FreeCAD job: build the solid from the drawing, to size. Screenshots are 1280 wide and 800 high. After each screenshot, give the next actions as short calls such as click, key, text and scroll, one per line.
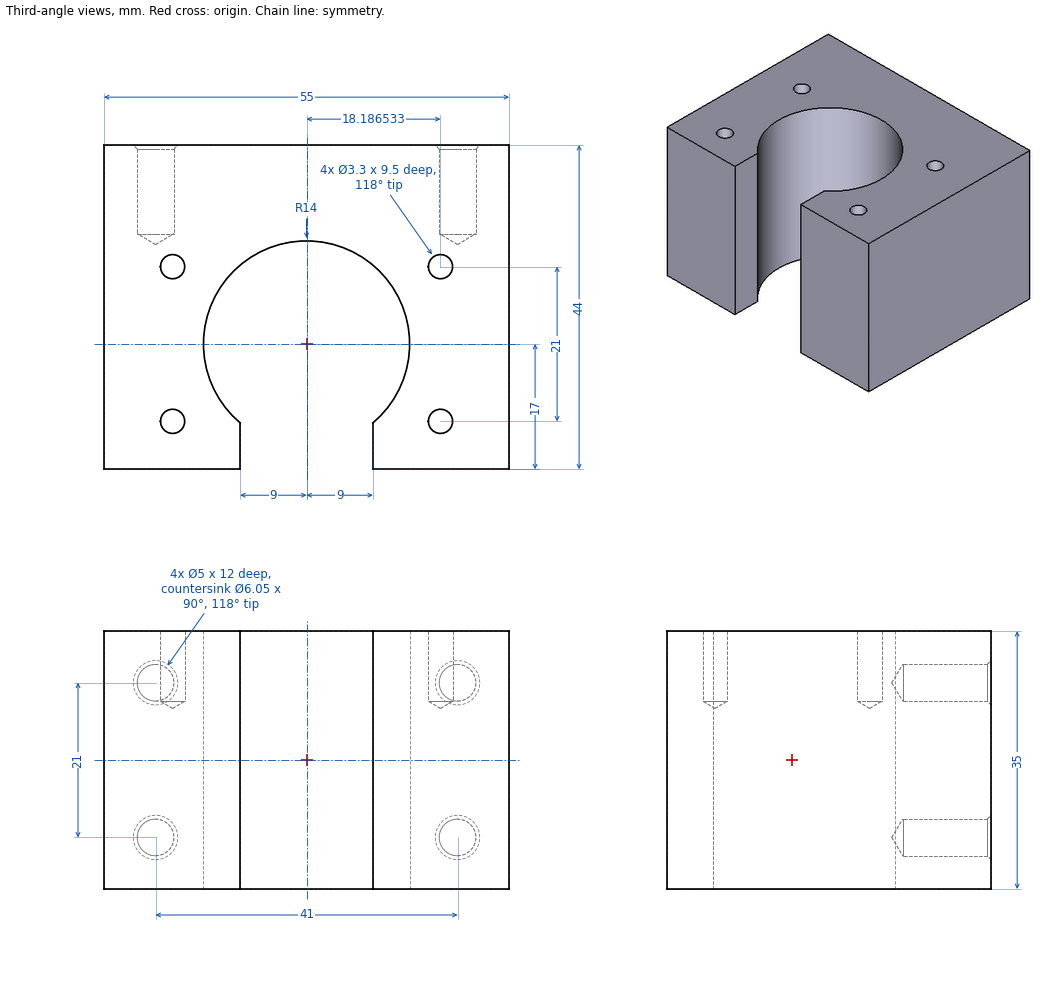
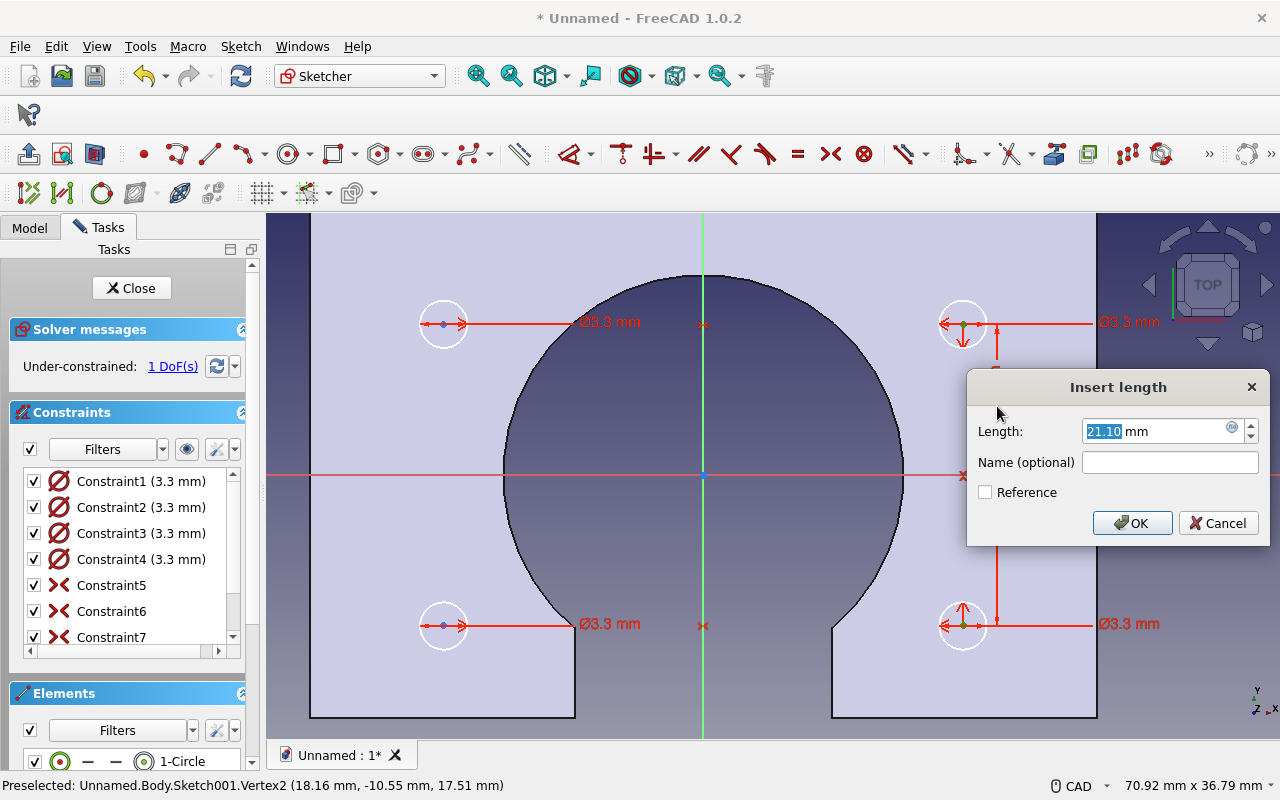
text(21)
key(Return)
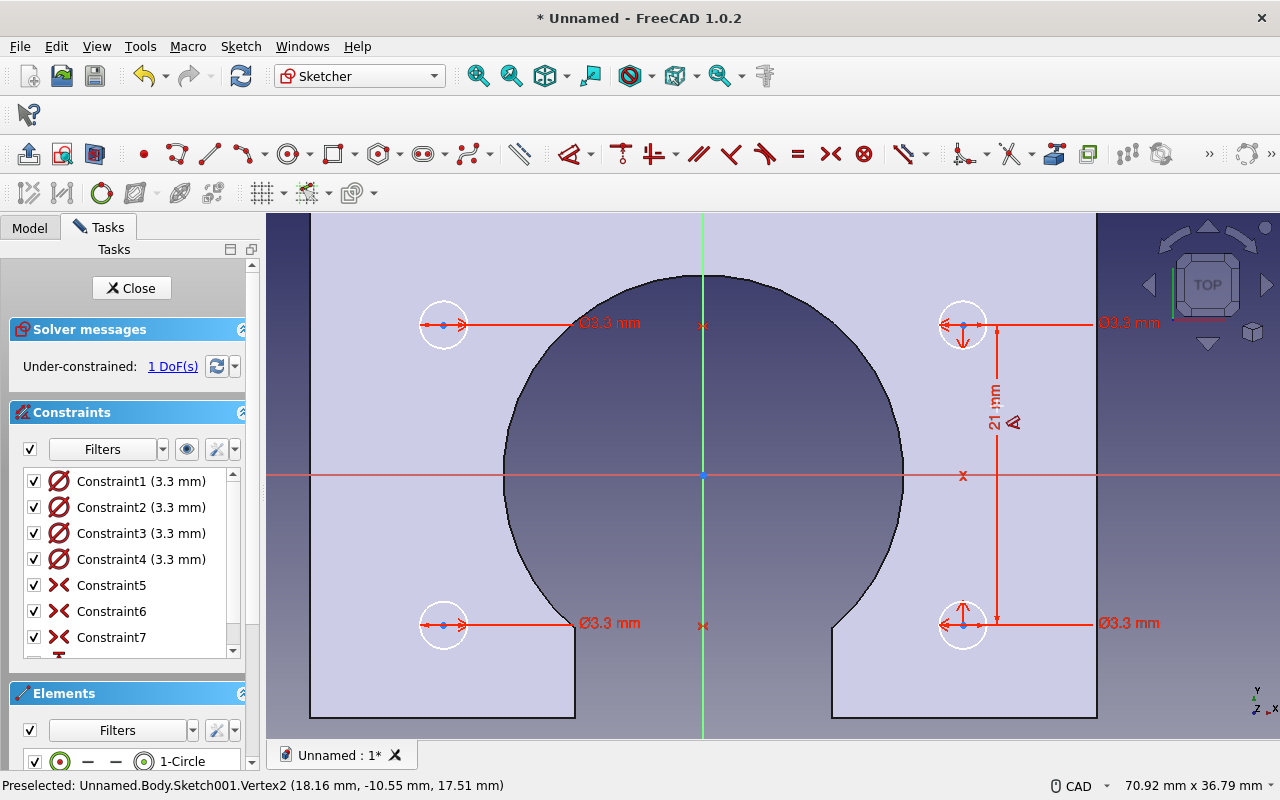
click(963, 325)
click(833, 291)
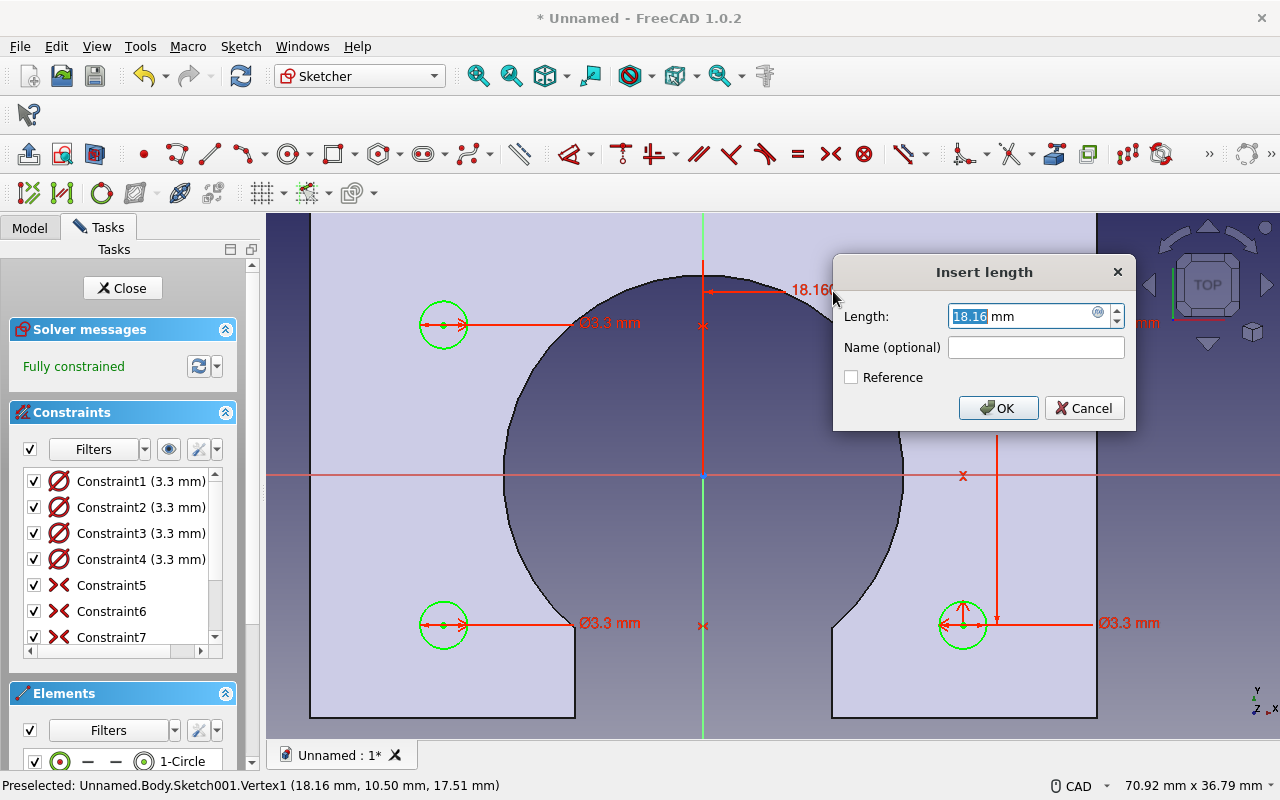
text(18.186533)
key(Return)
key(Escape)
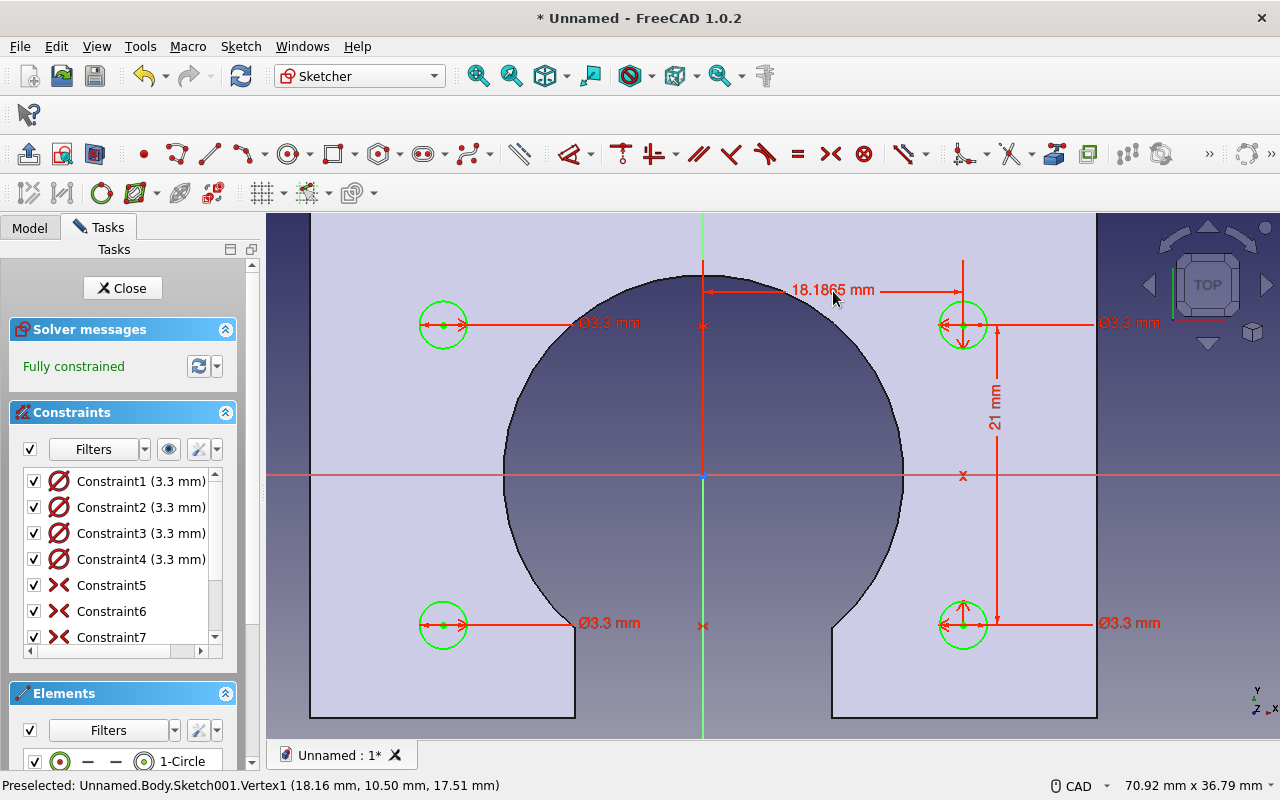
click(123, 288)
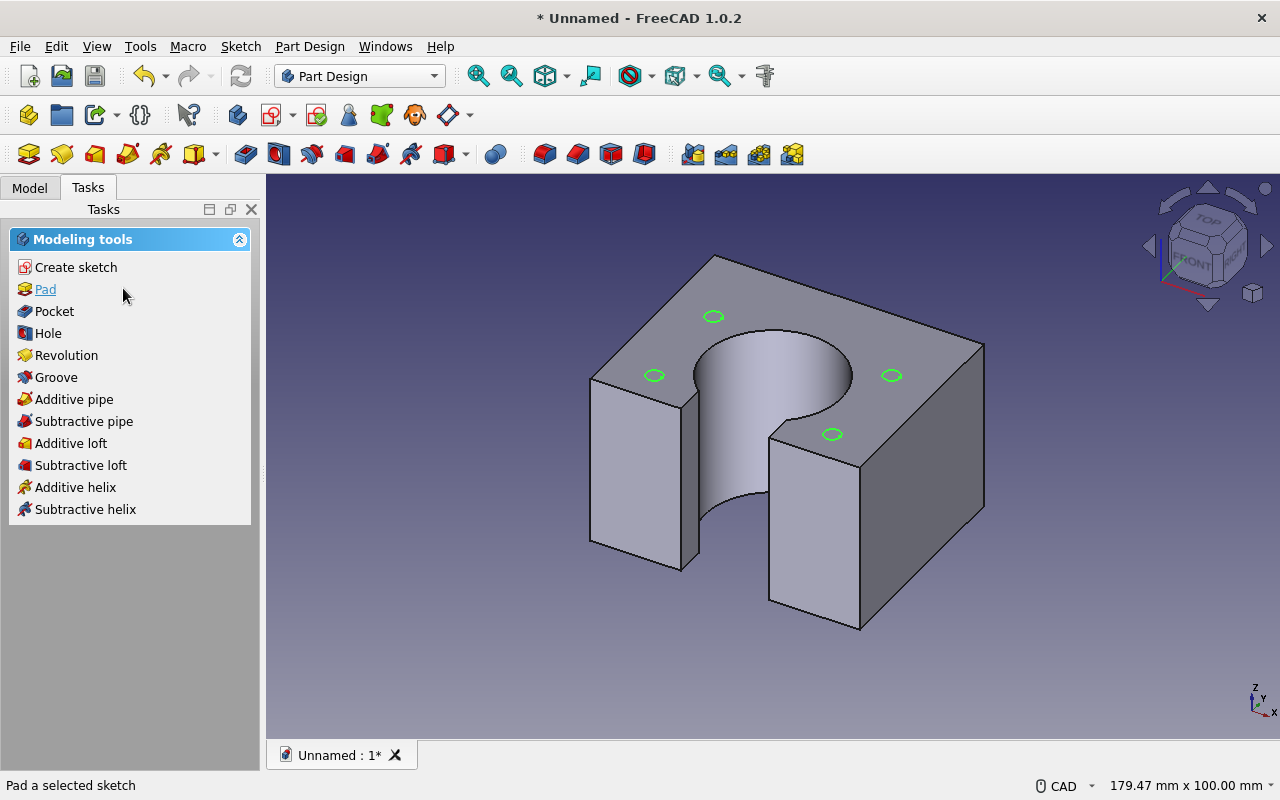
click(279, 154)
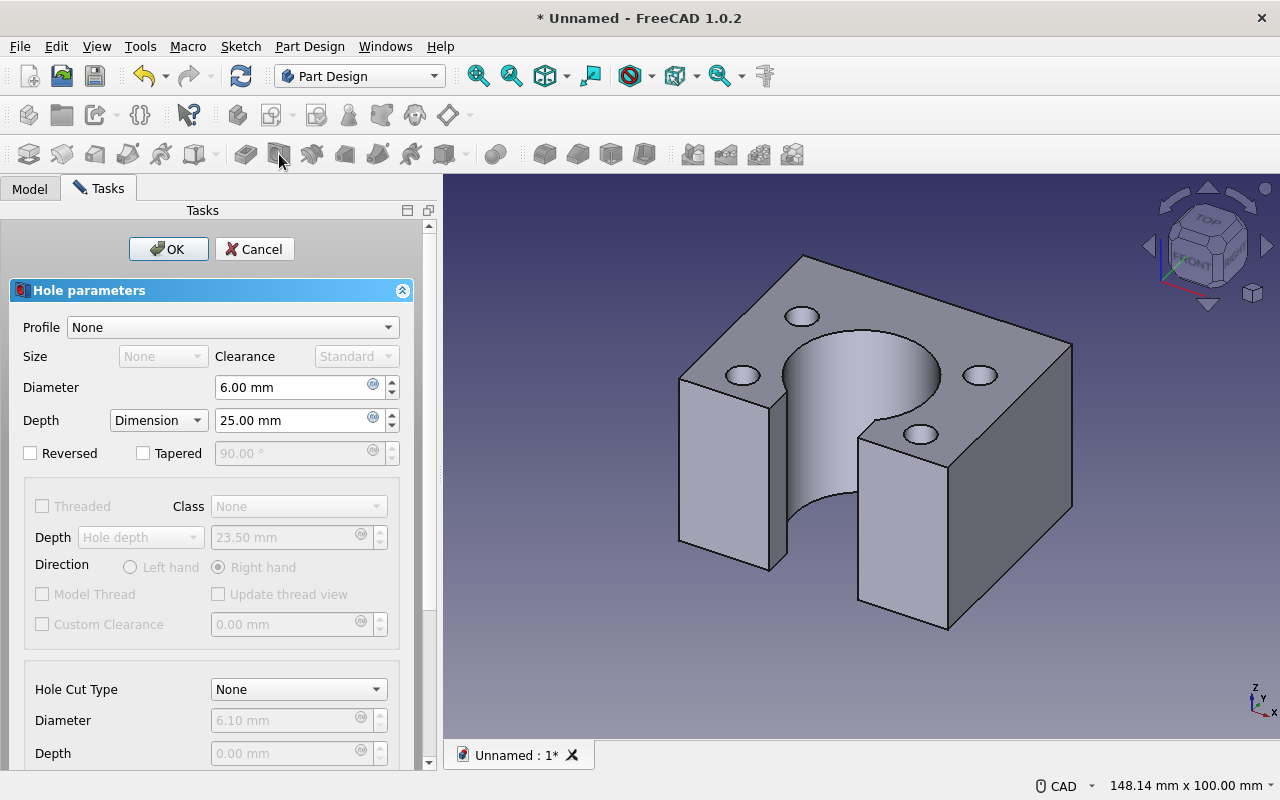
triple_click(300, 388)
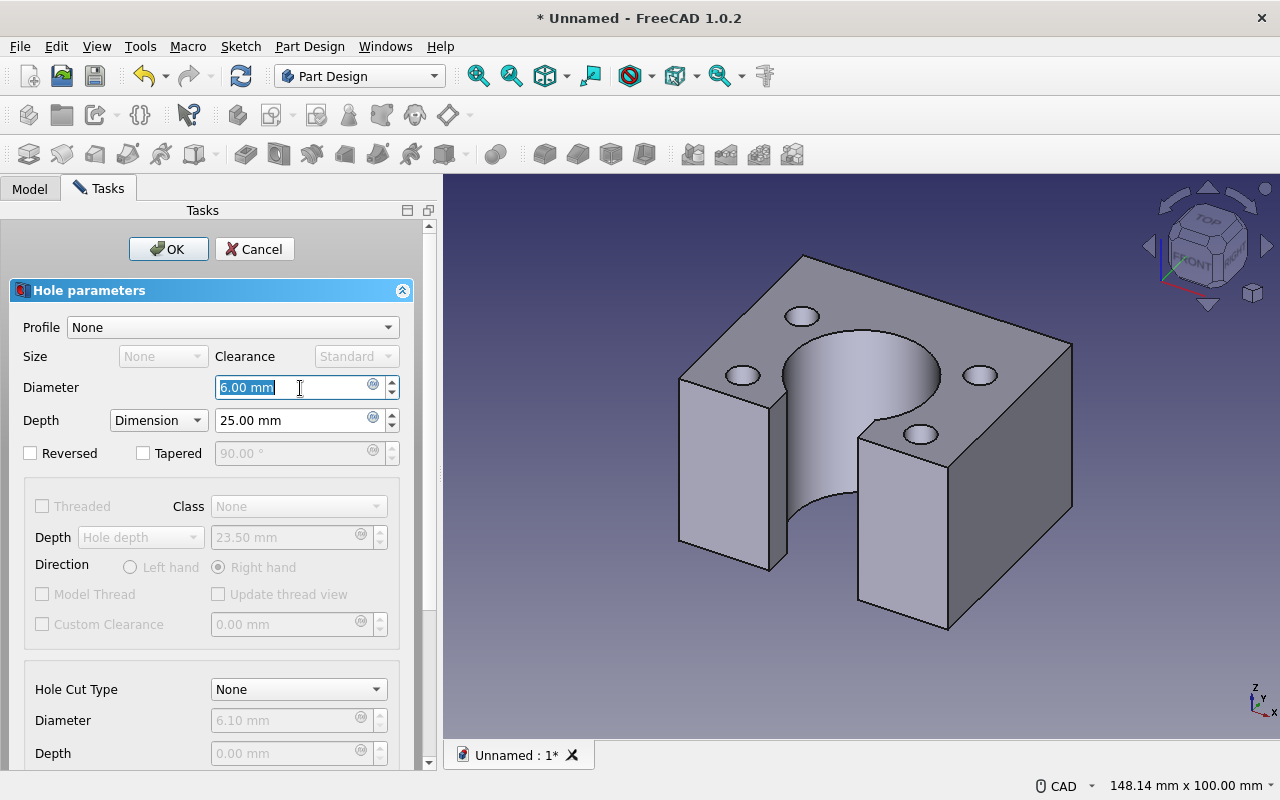
text(3.3)
key(Tab)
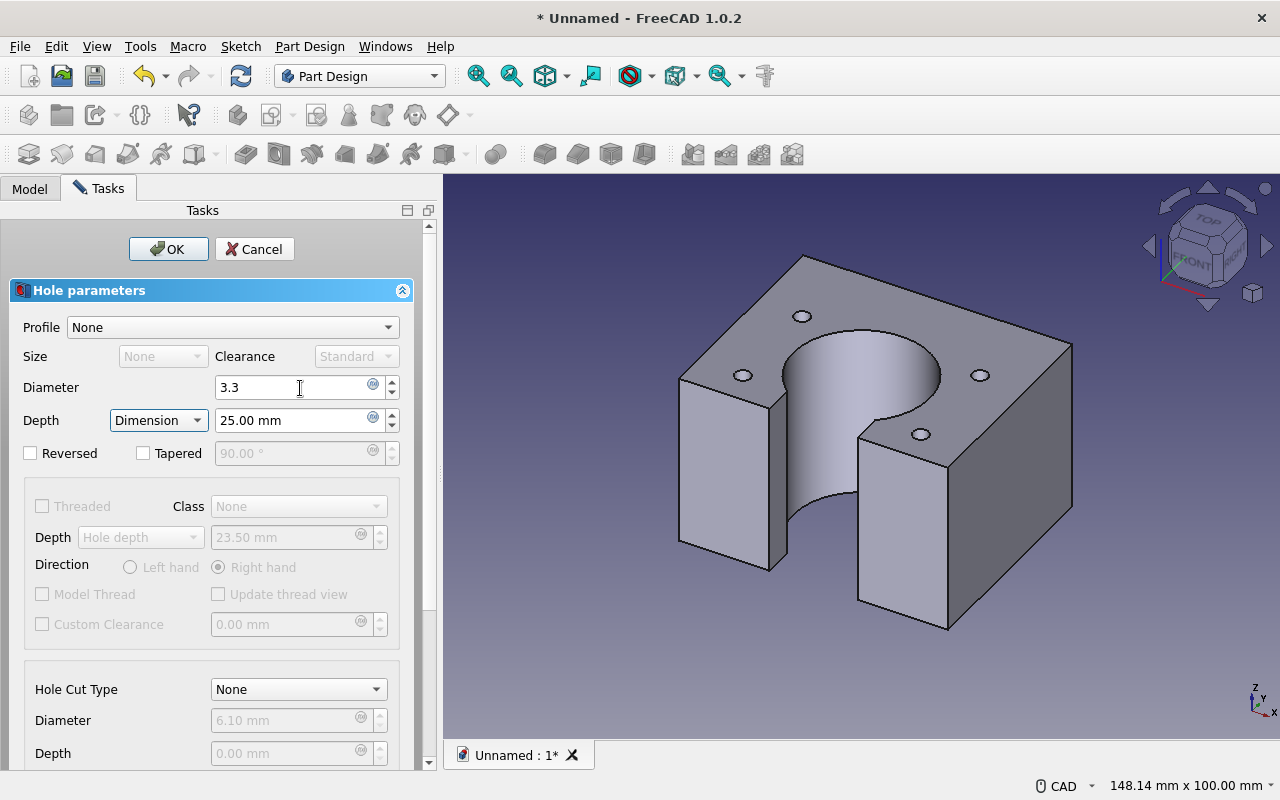
triple_click(300, 420)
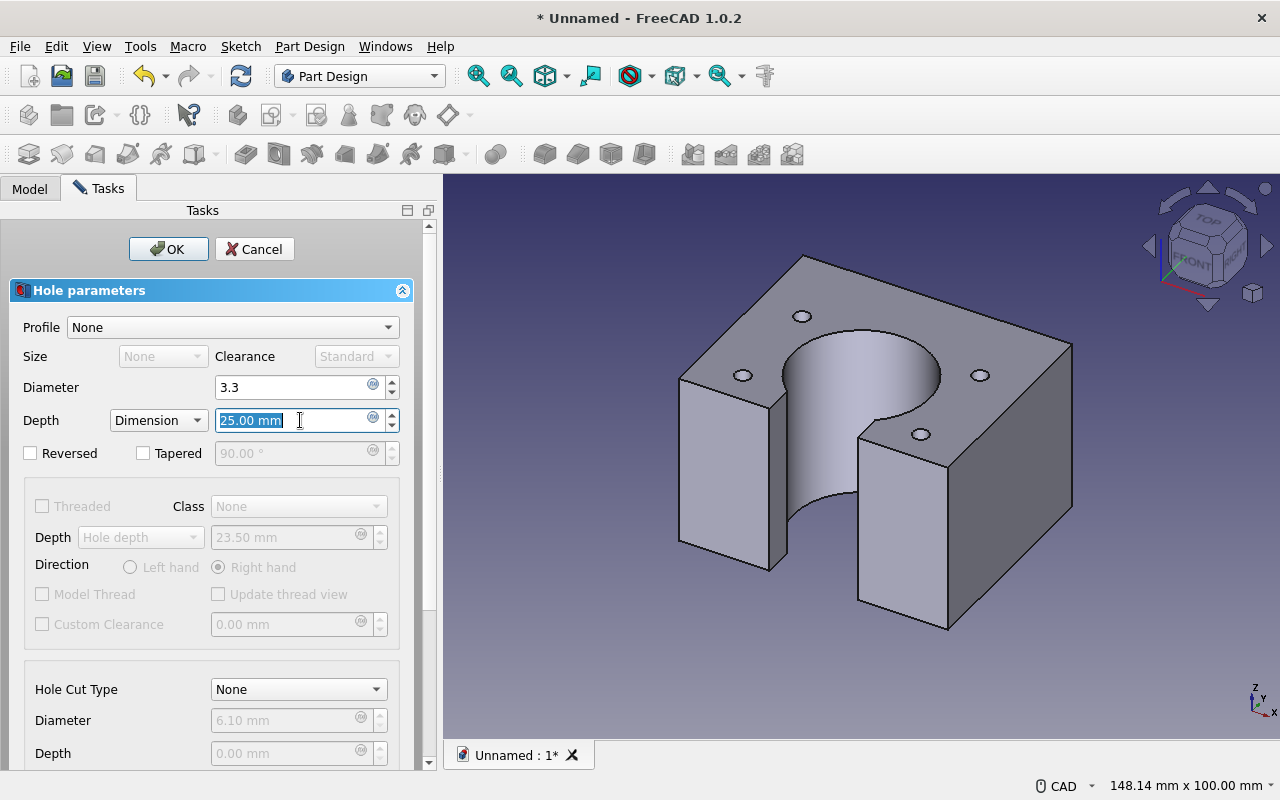
text(9.5)
key(Tab)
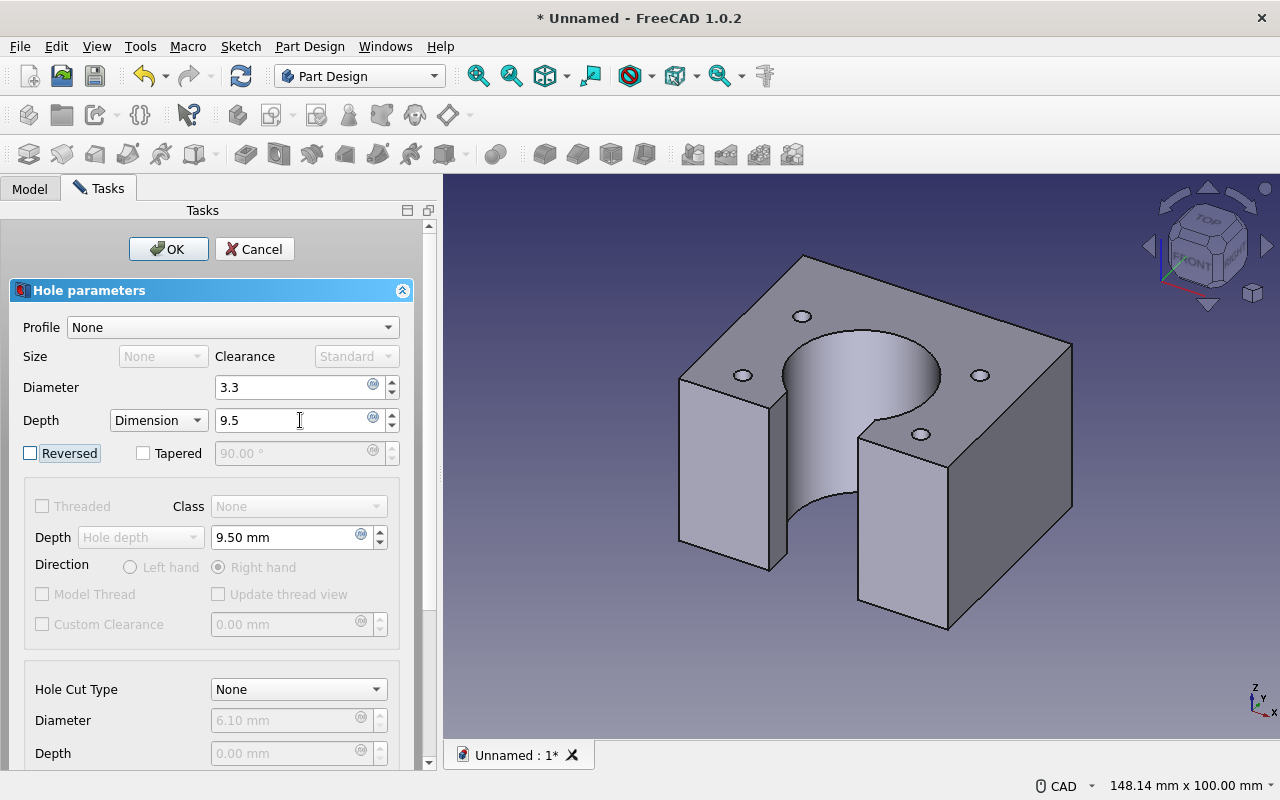
click(169, 249)